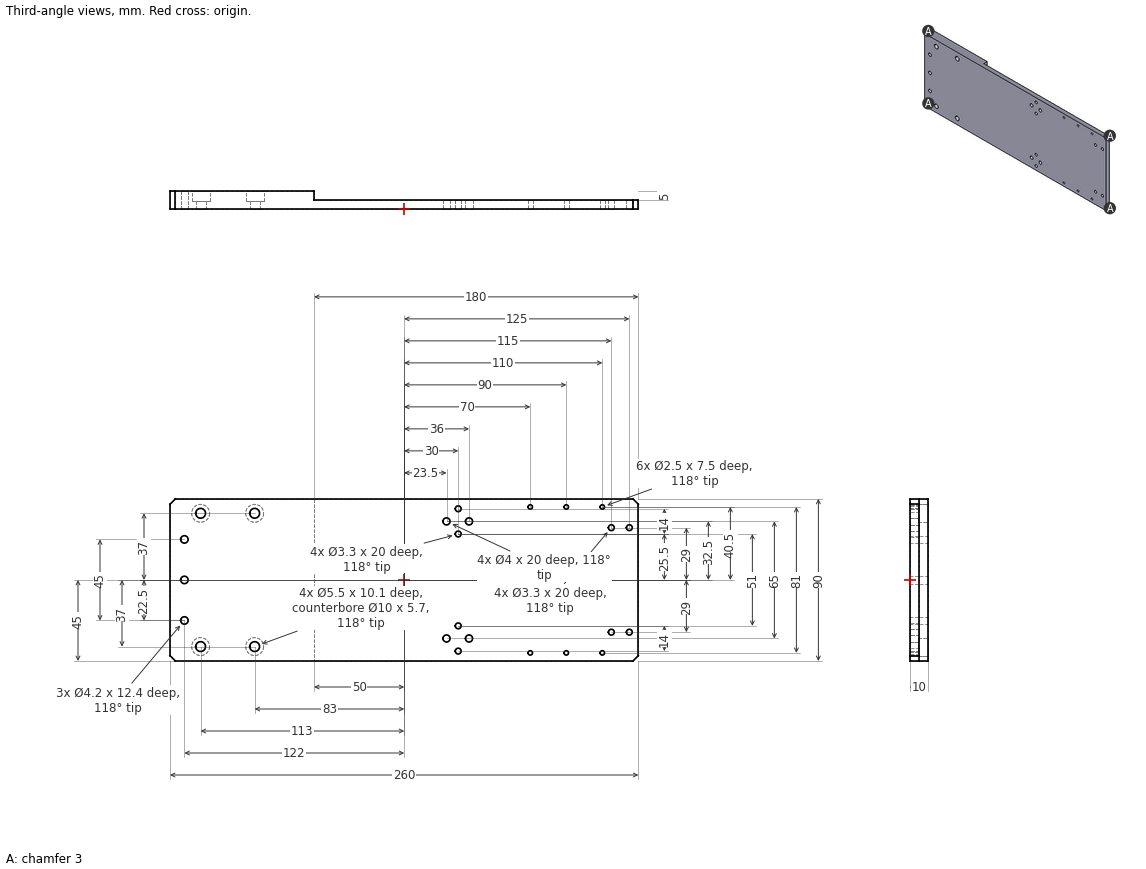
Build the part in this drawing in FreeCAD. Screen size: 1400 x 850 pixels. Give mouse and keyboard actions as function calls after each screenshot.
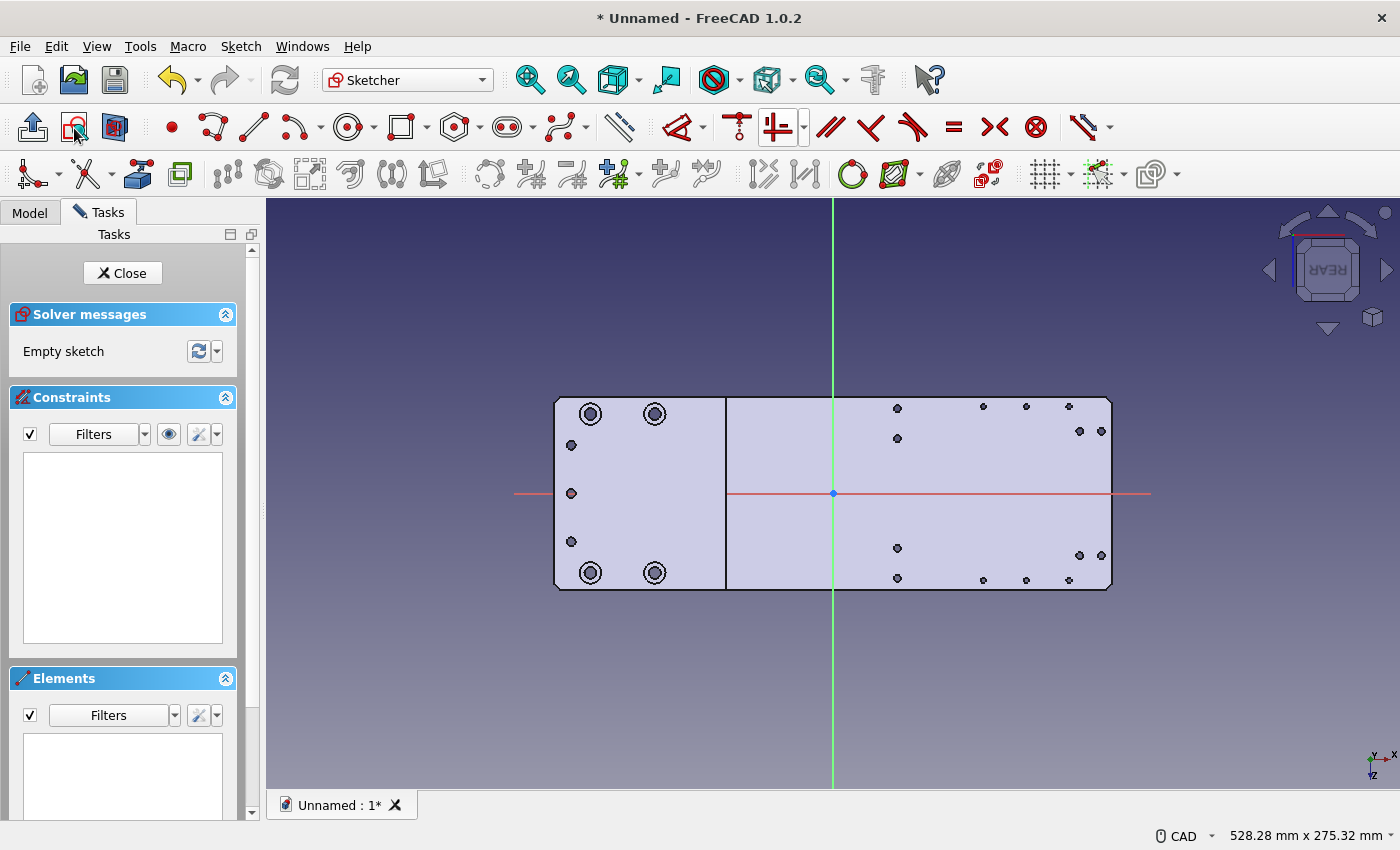
scroll(937, 493, up, 5)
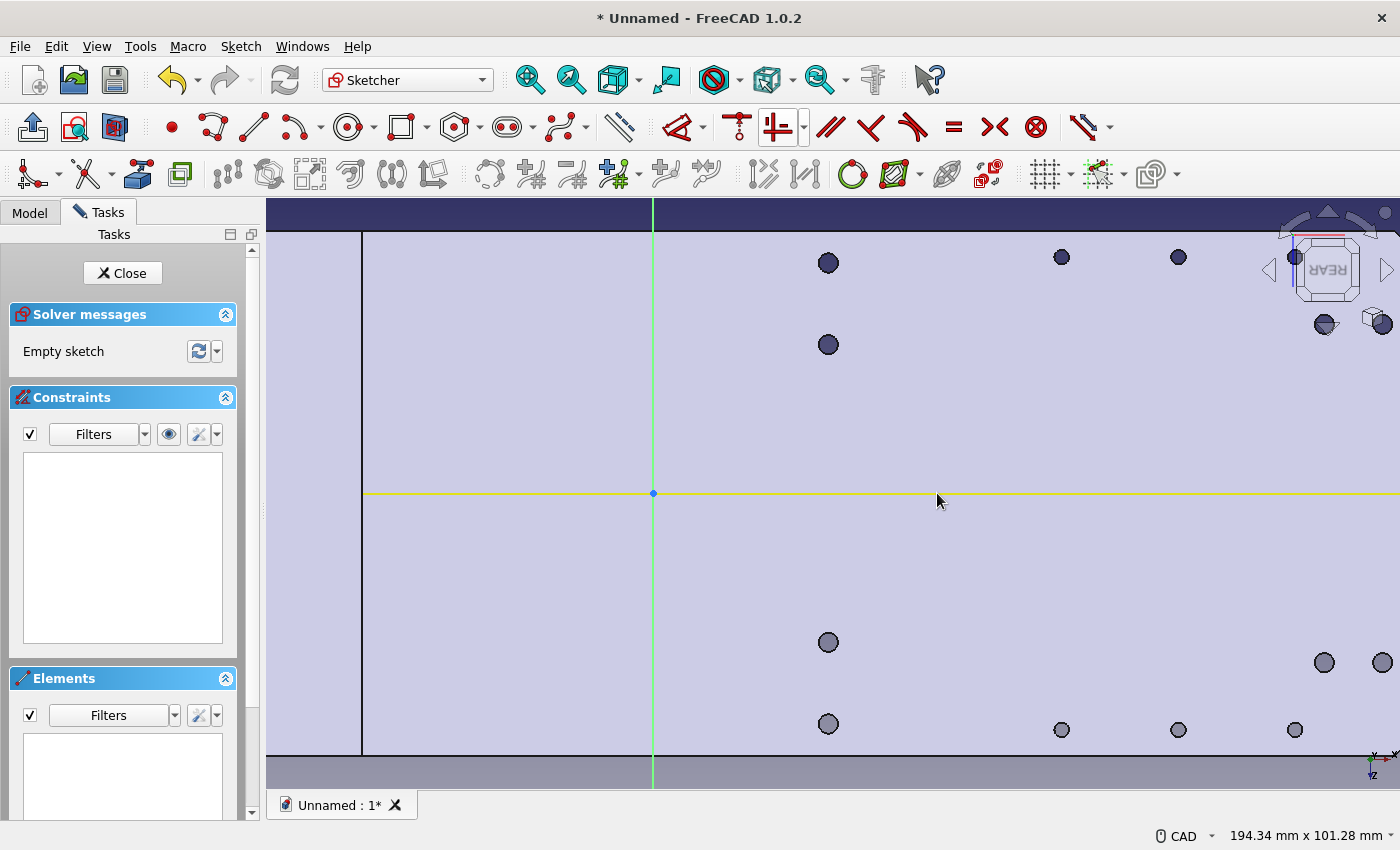
click(348, 128)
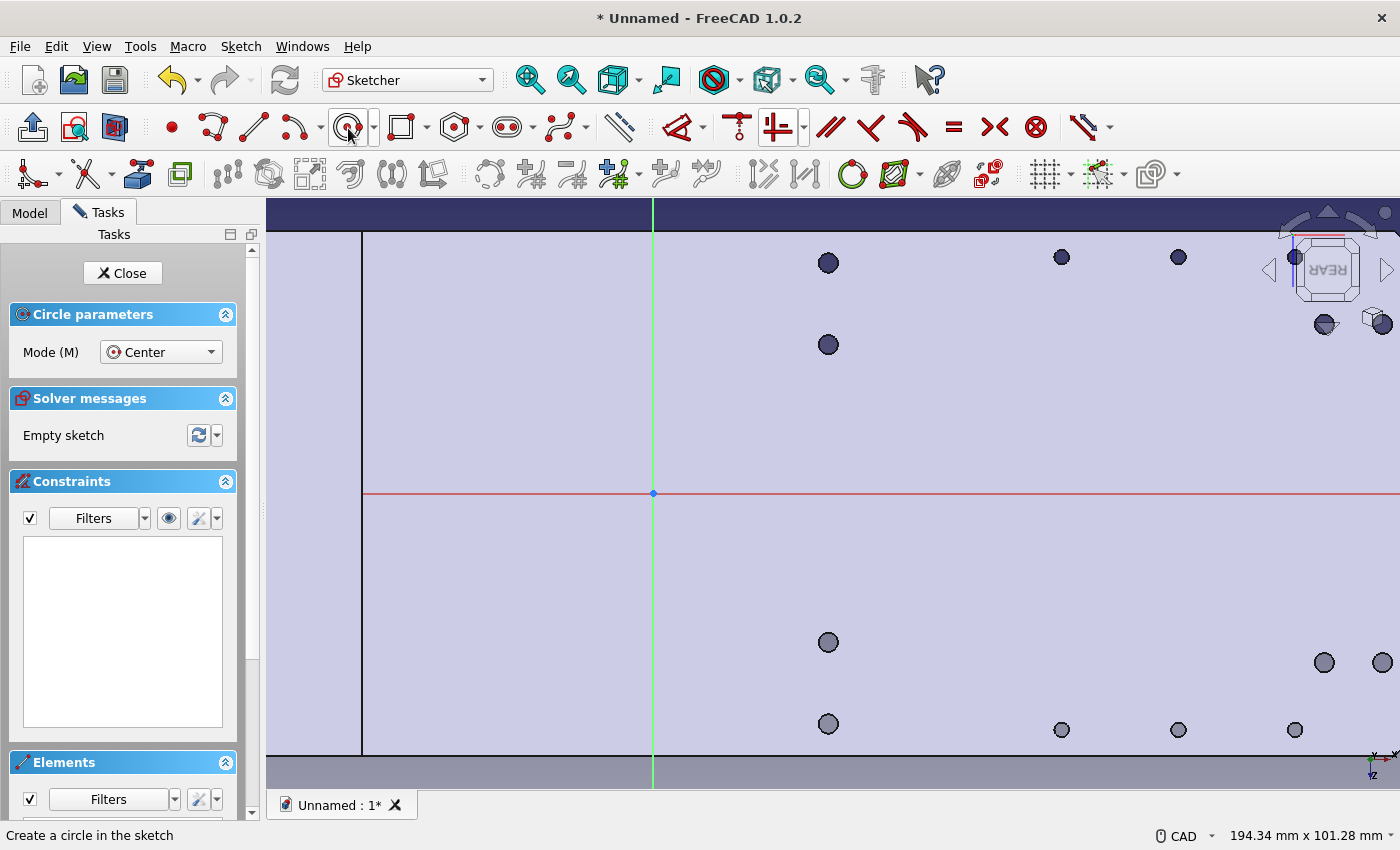
scroll(790, 683, up, 4)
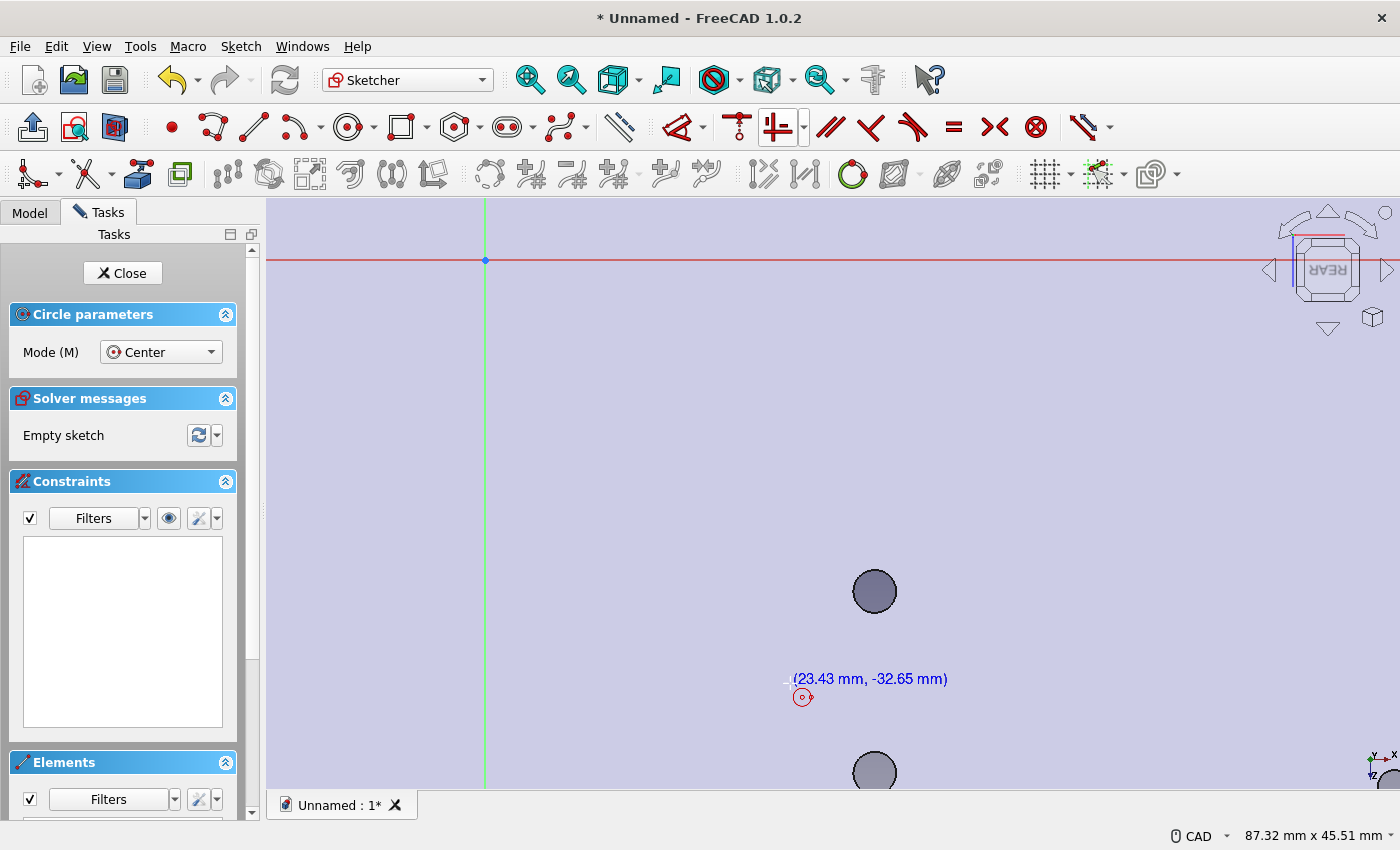
click(790, 682)
click(809, 664)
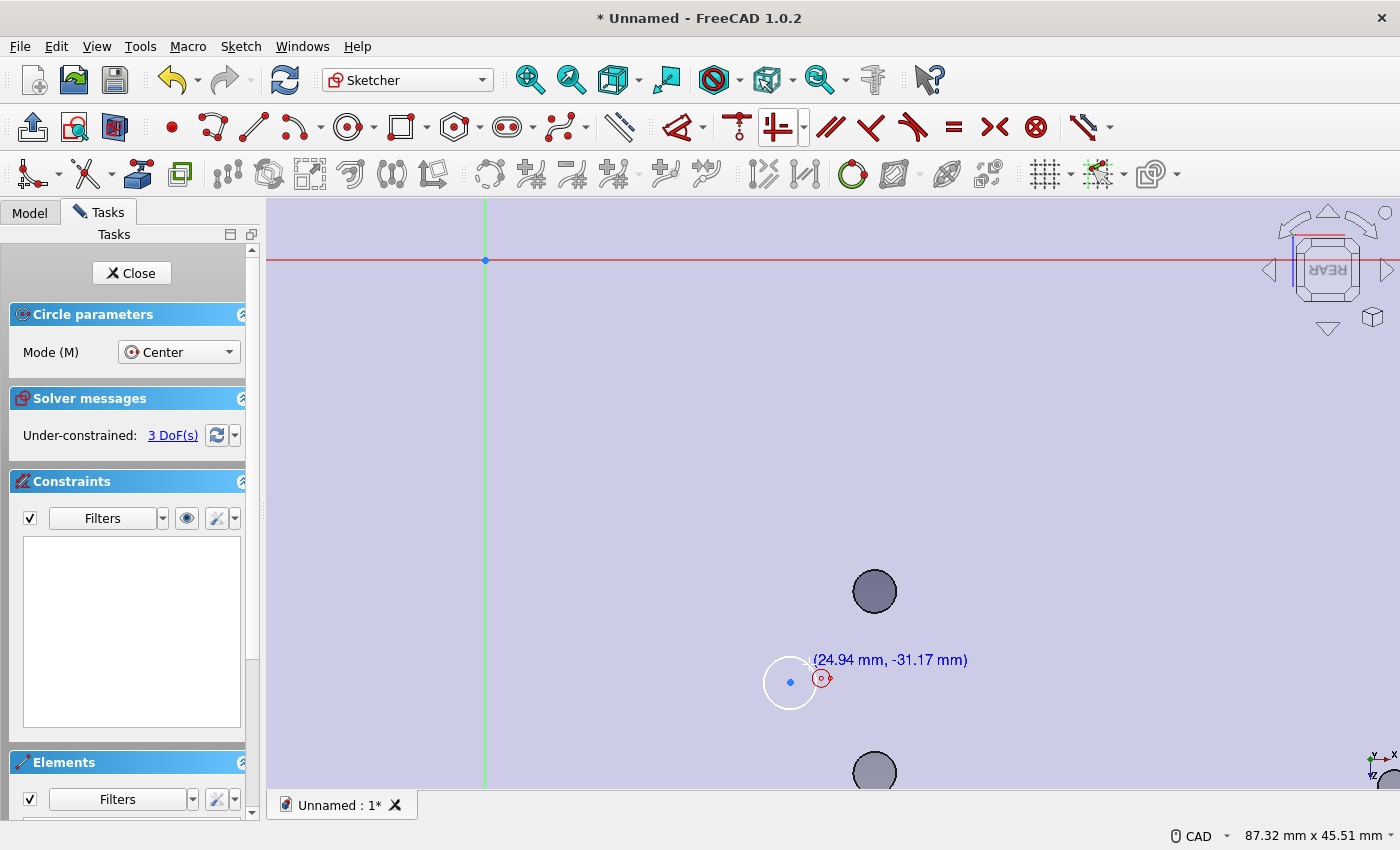
click(953, 682)
click(971, 664)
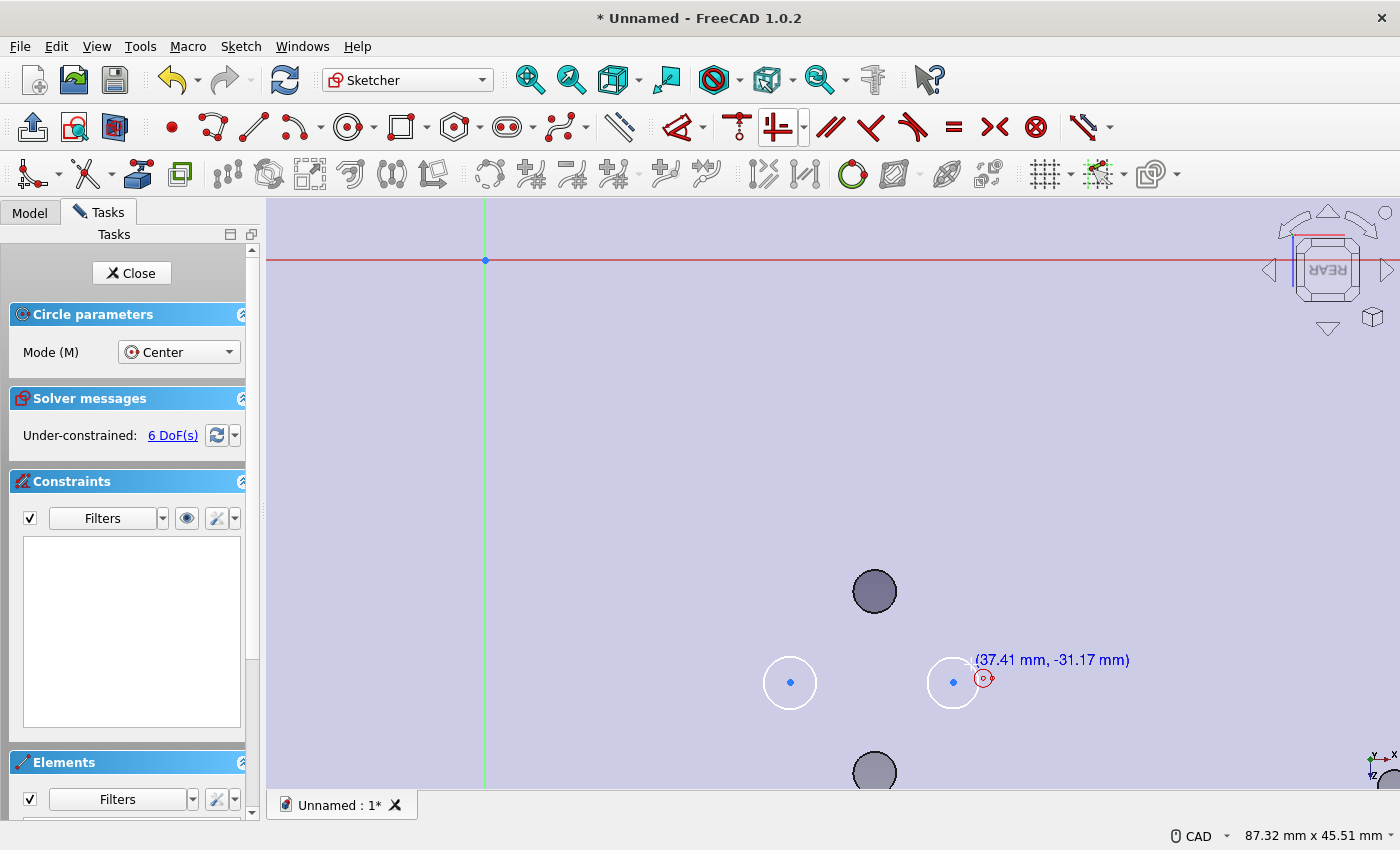
scroll(791, 684, down, 4)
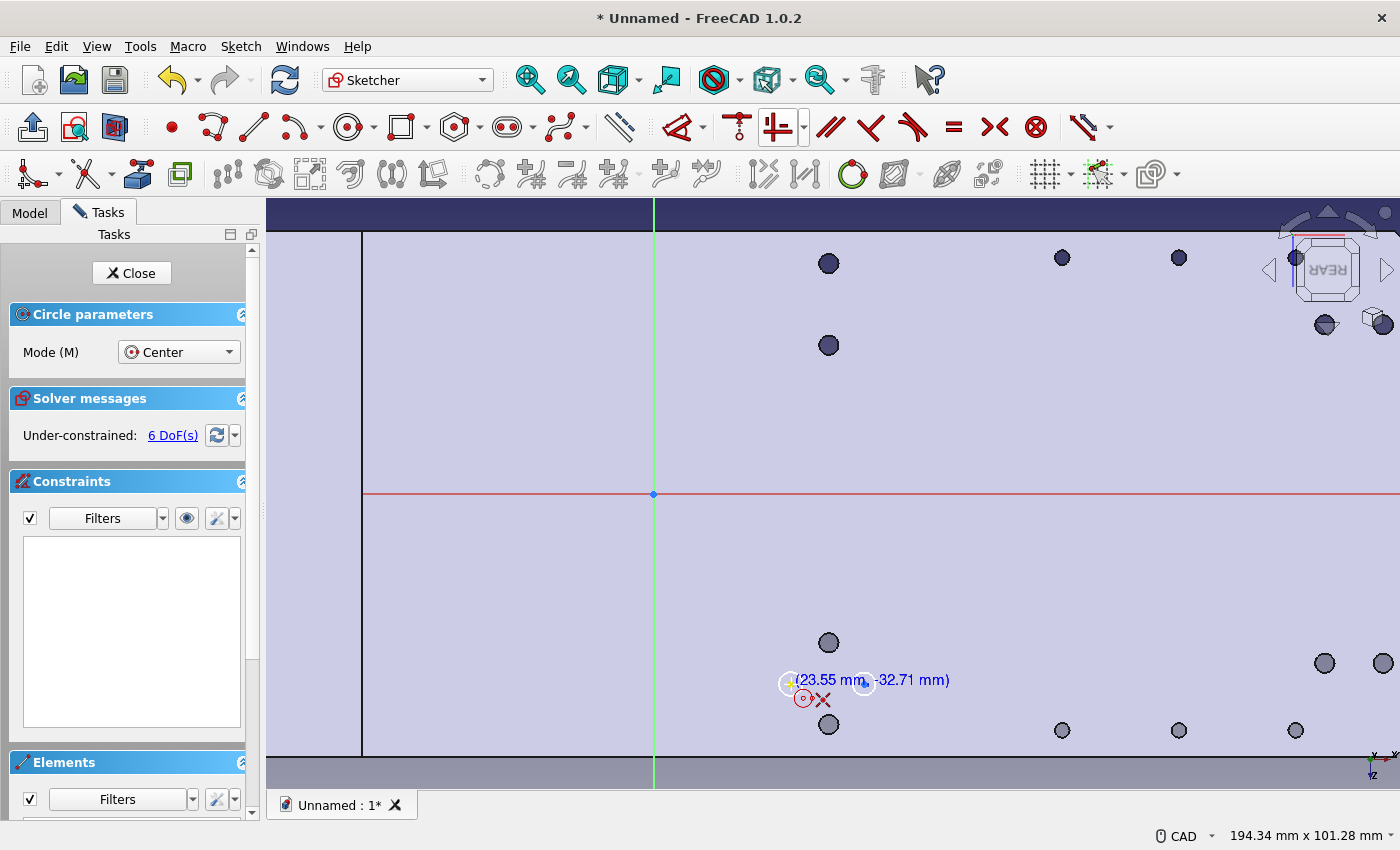
scroll(791, 304, up, 4)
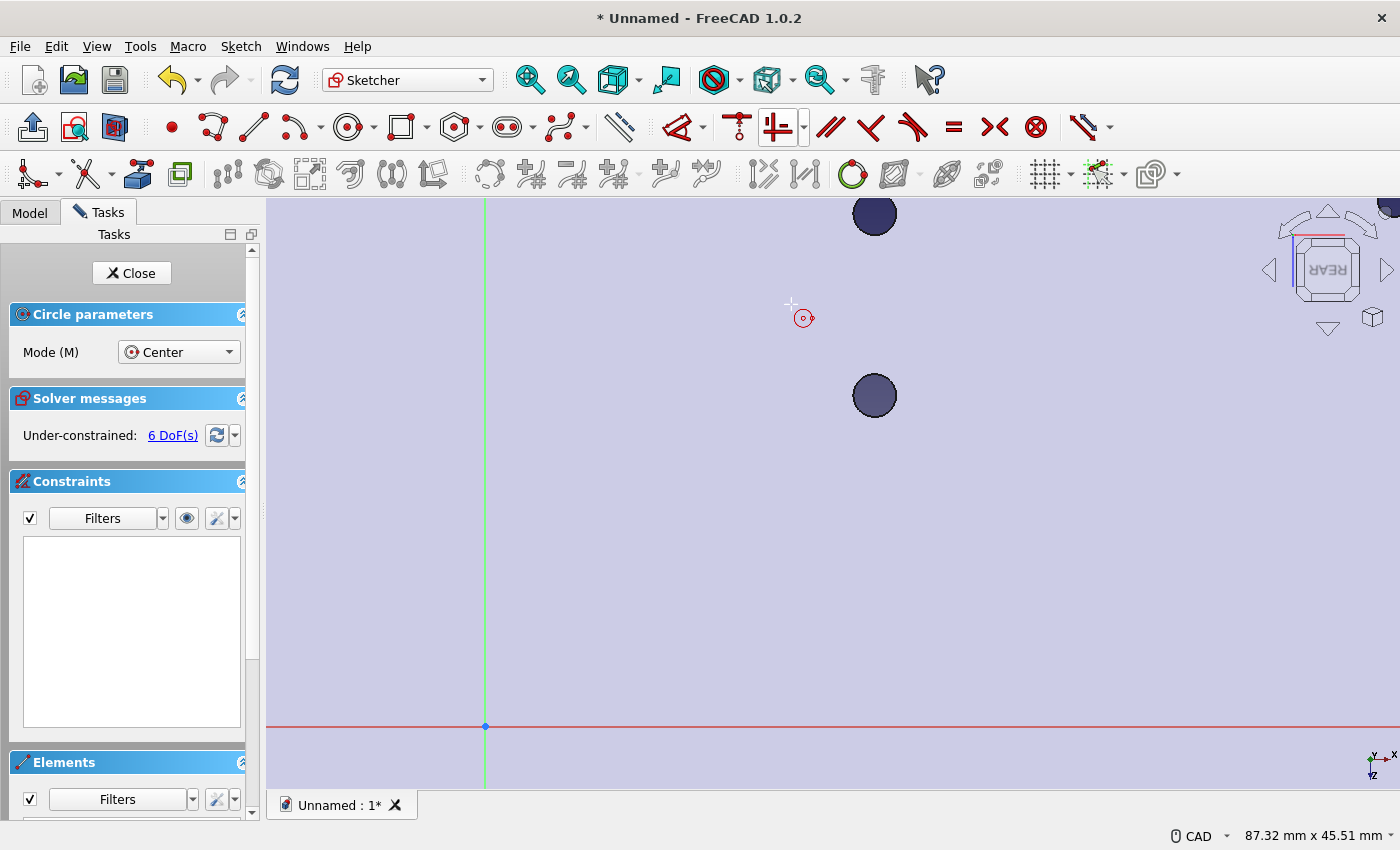
click(790, 305)
click(809, 286)